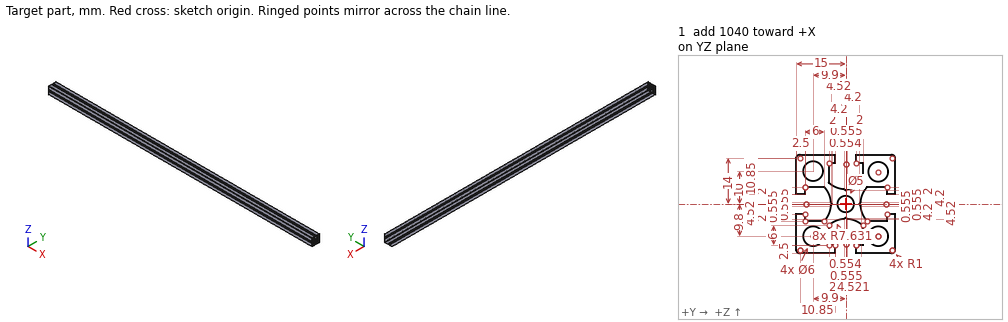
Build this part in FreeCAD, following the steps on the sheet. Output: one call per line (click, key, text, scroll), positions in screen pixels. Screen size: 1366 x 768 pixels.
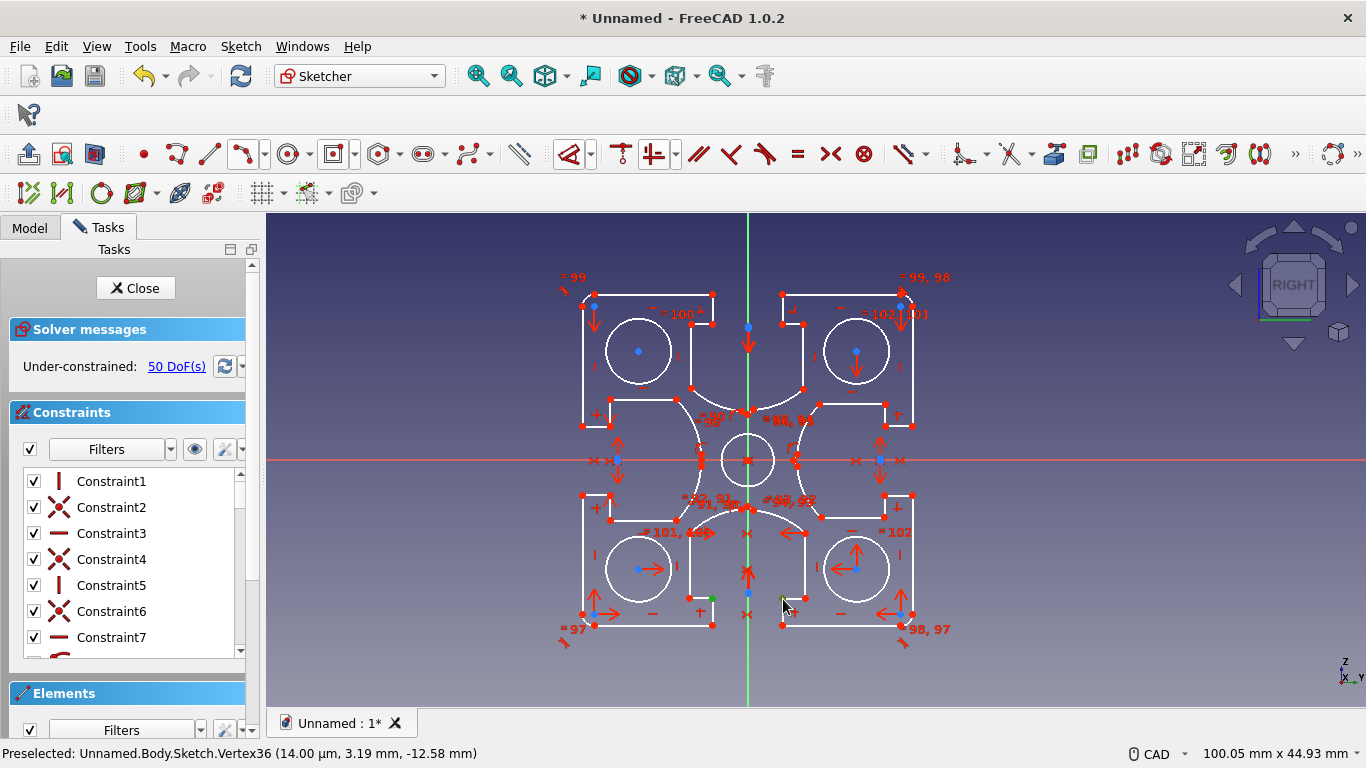
click(748, 648)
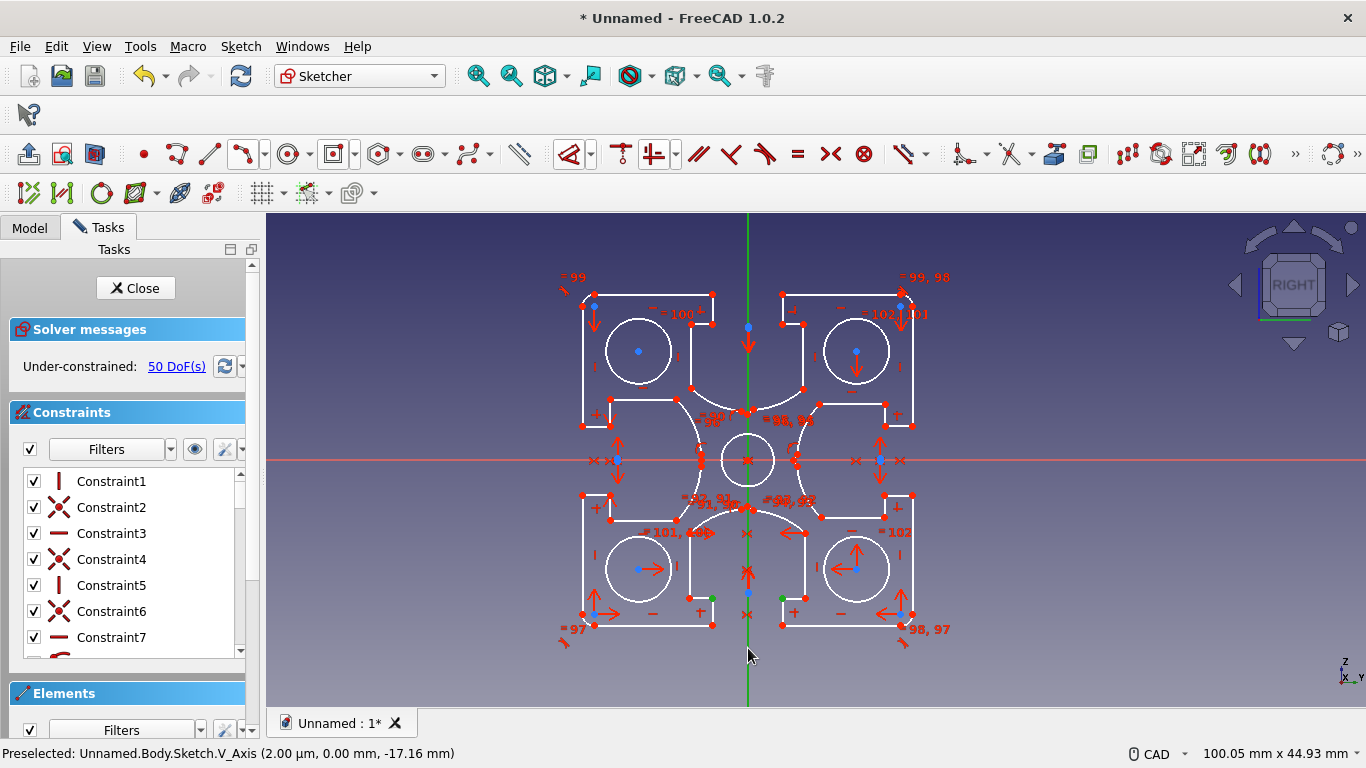
key(s)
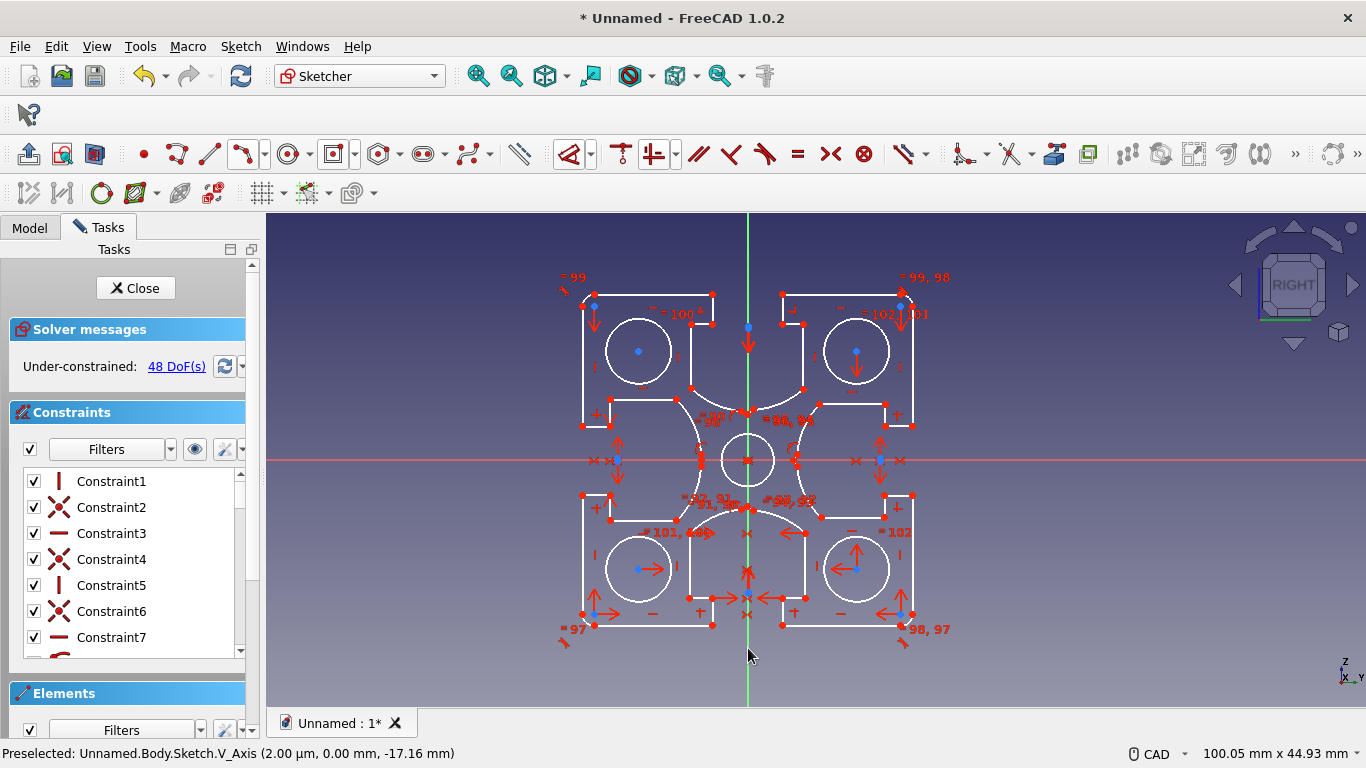
click(610, 495)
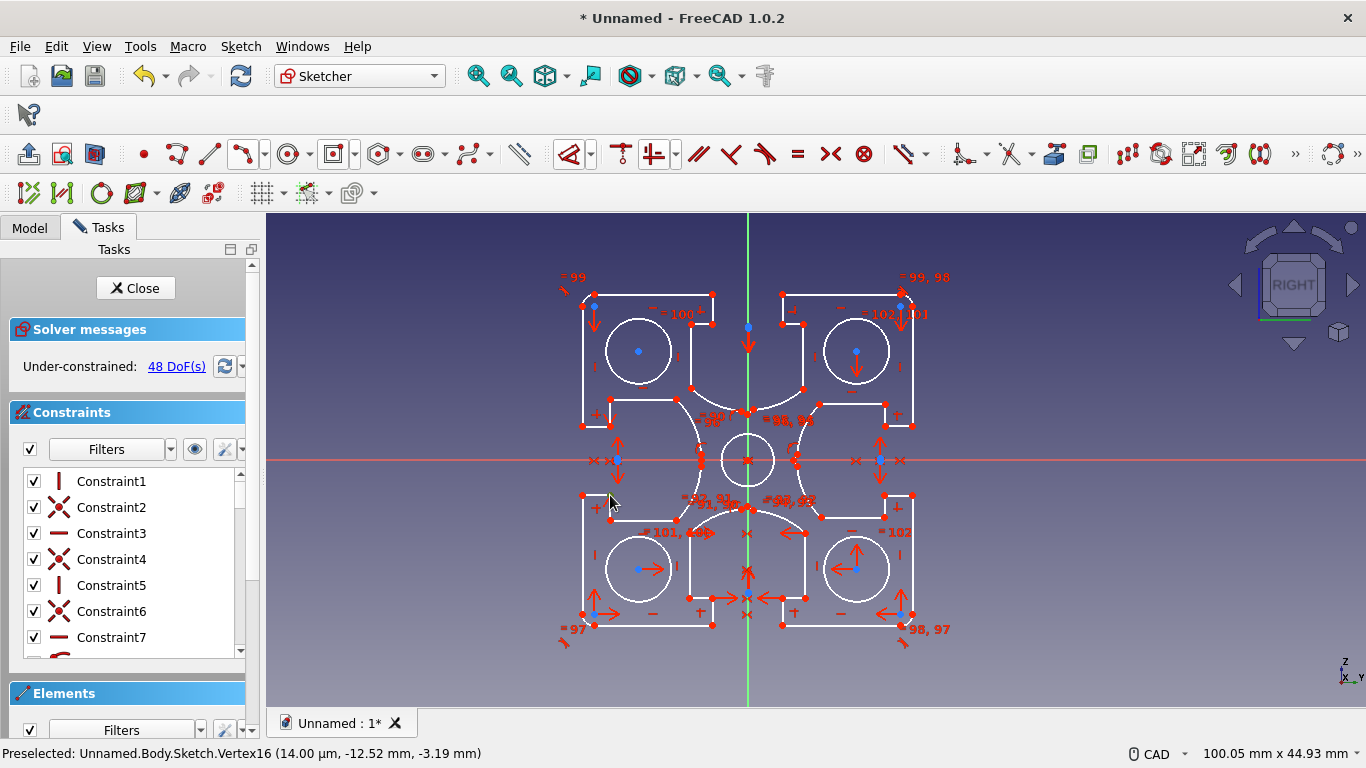
click(885, 496)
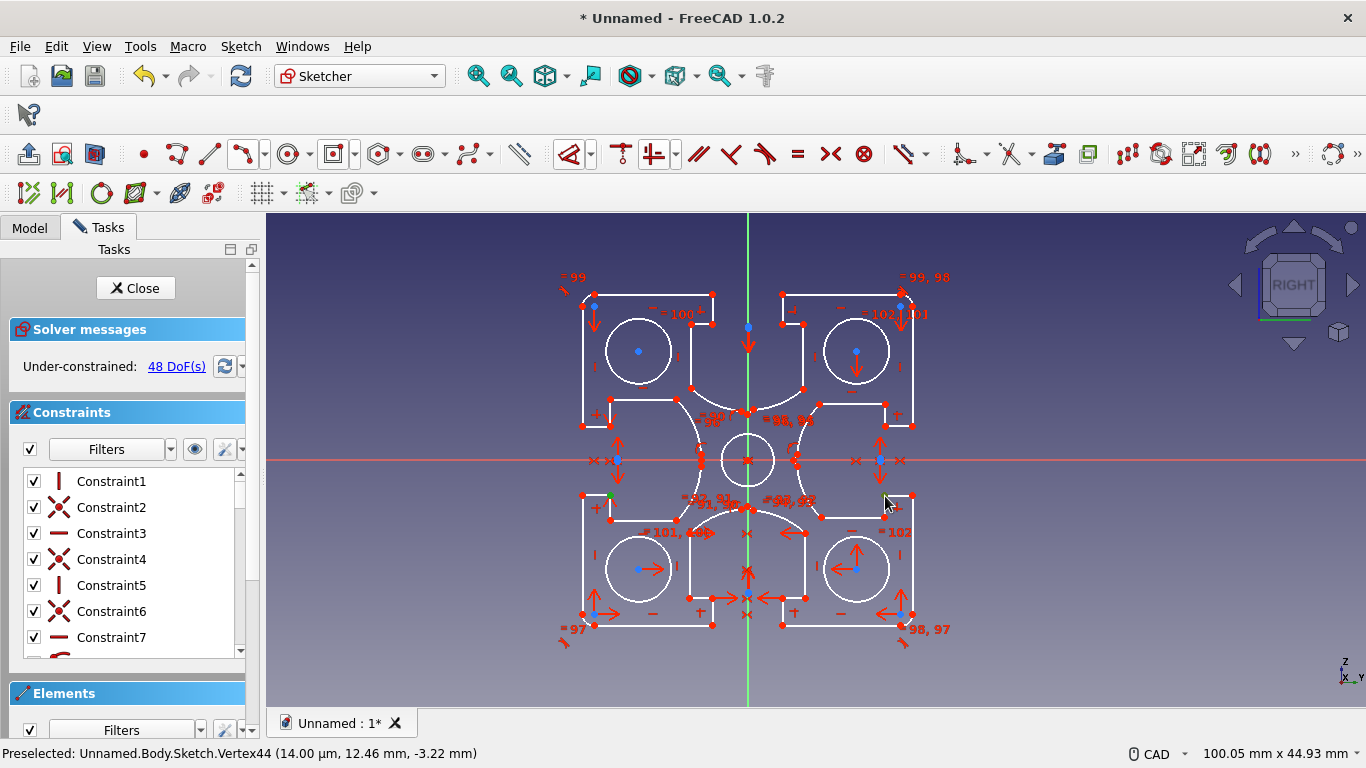
click(748, 648)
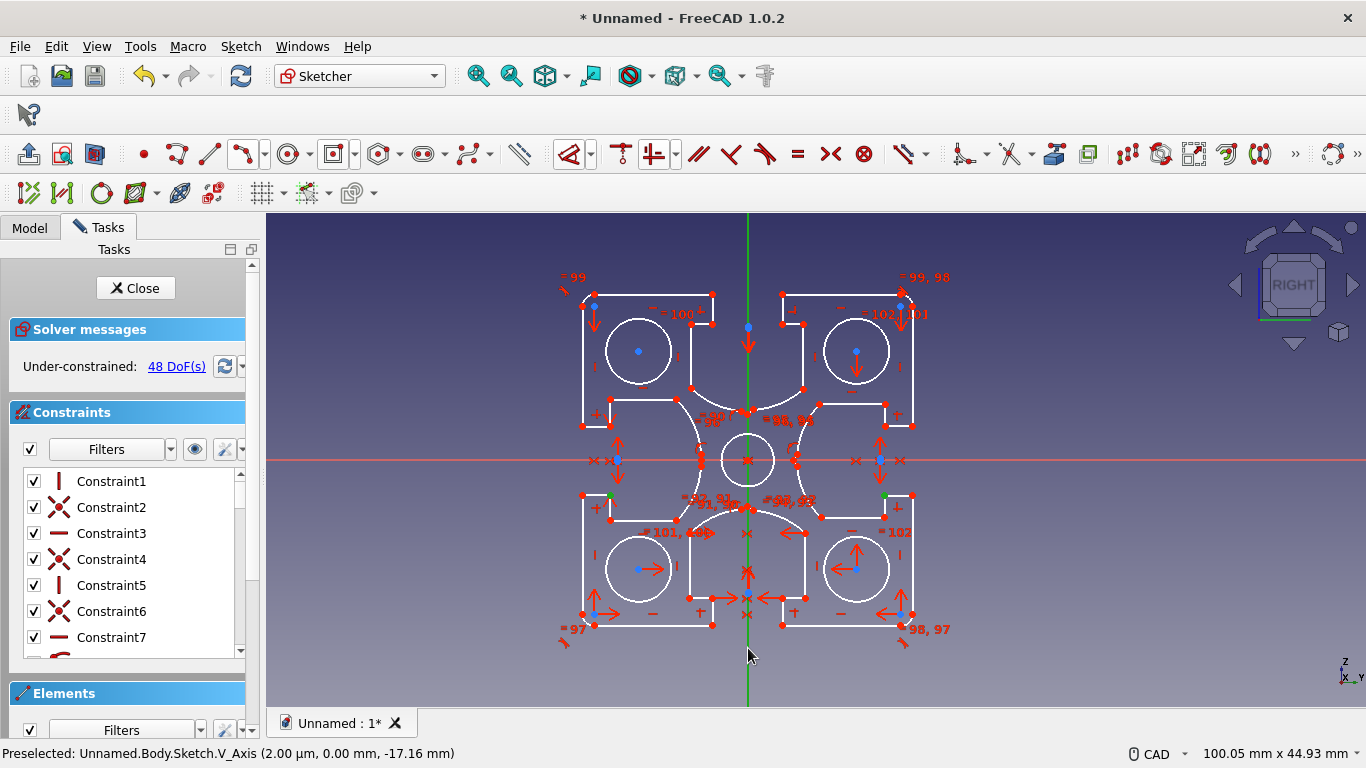
click(831, 154)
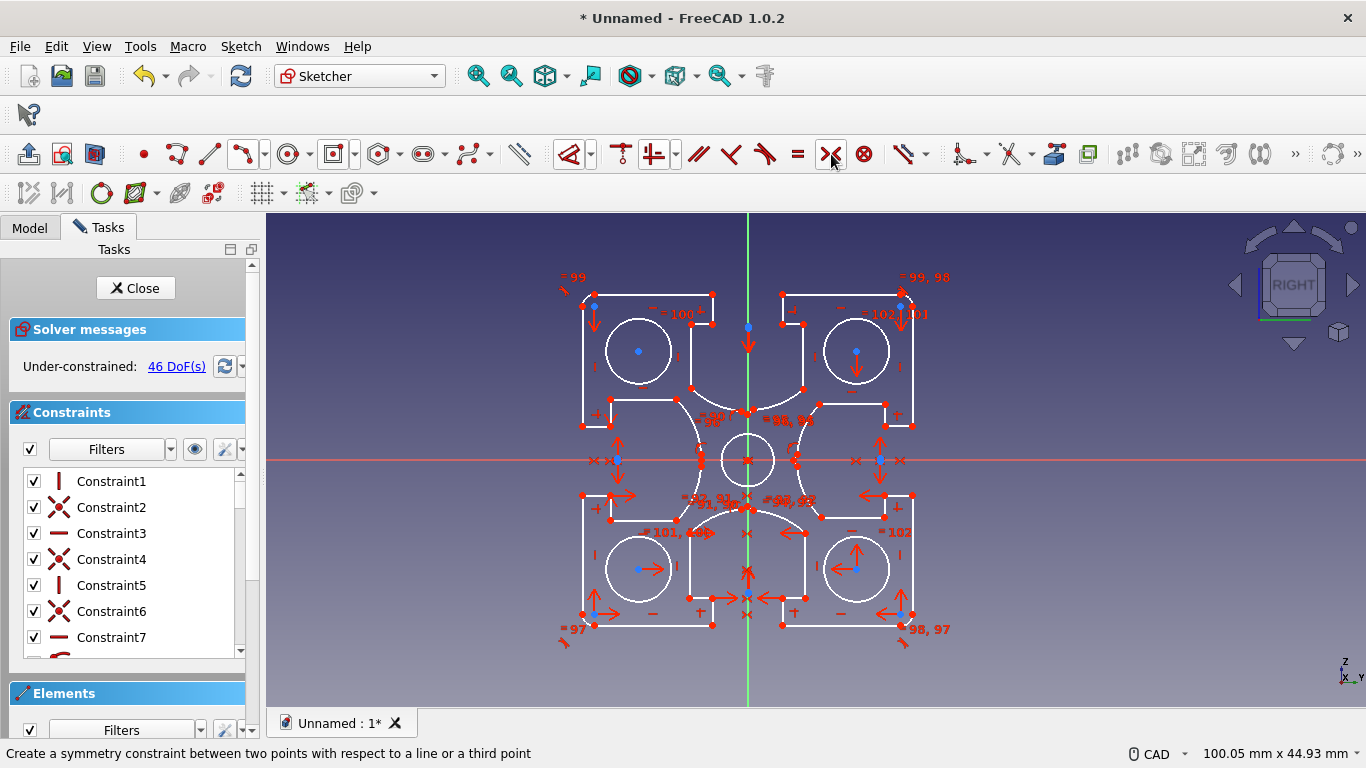
click(677, 521)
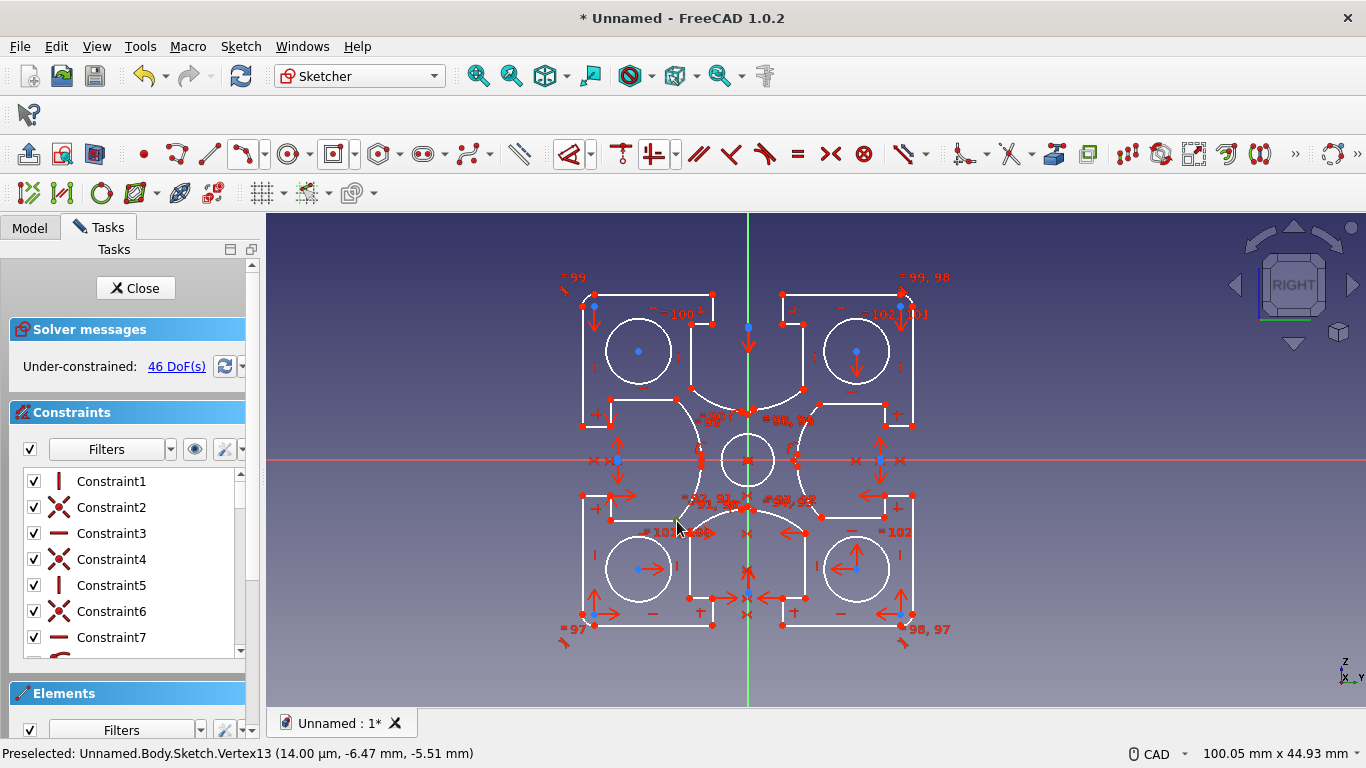
click(821, 518)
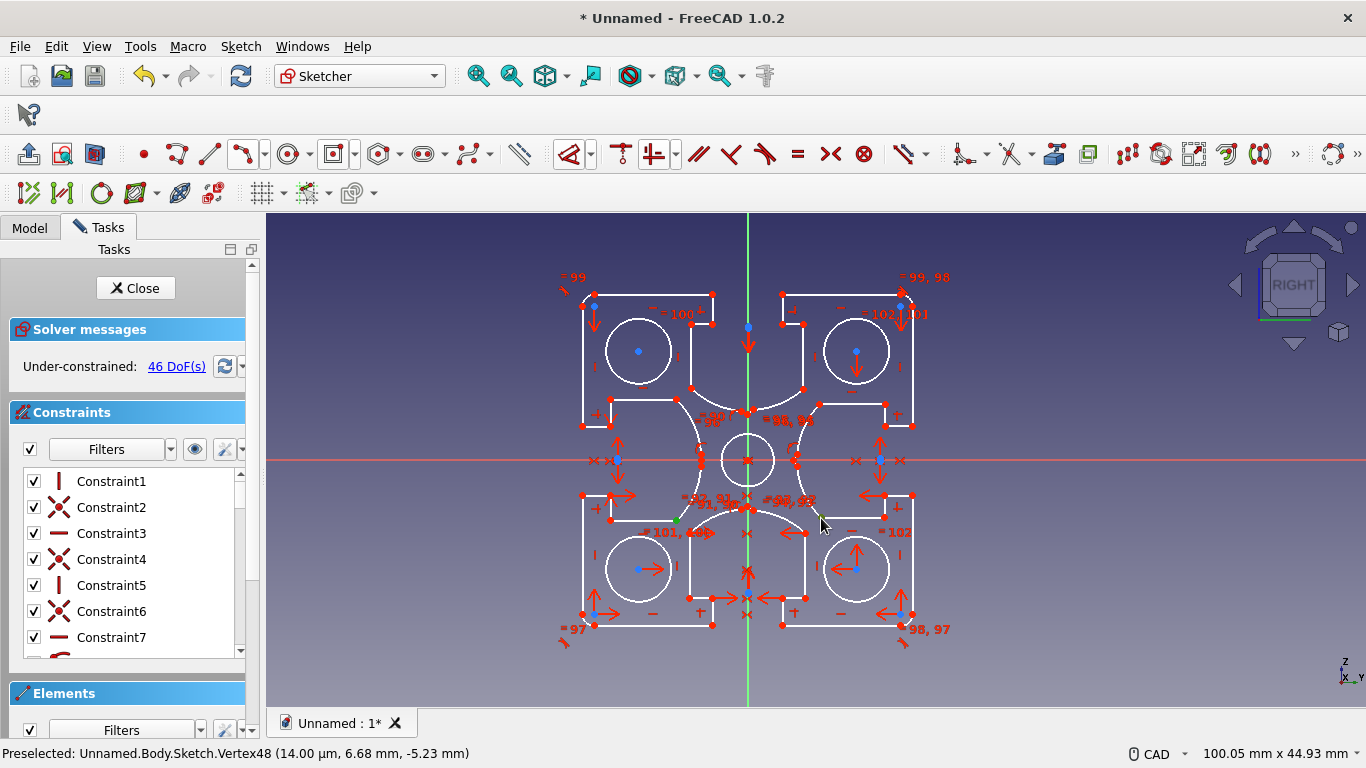
click(748, 648)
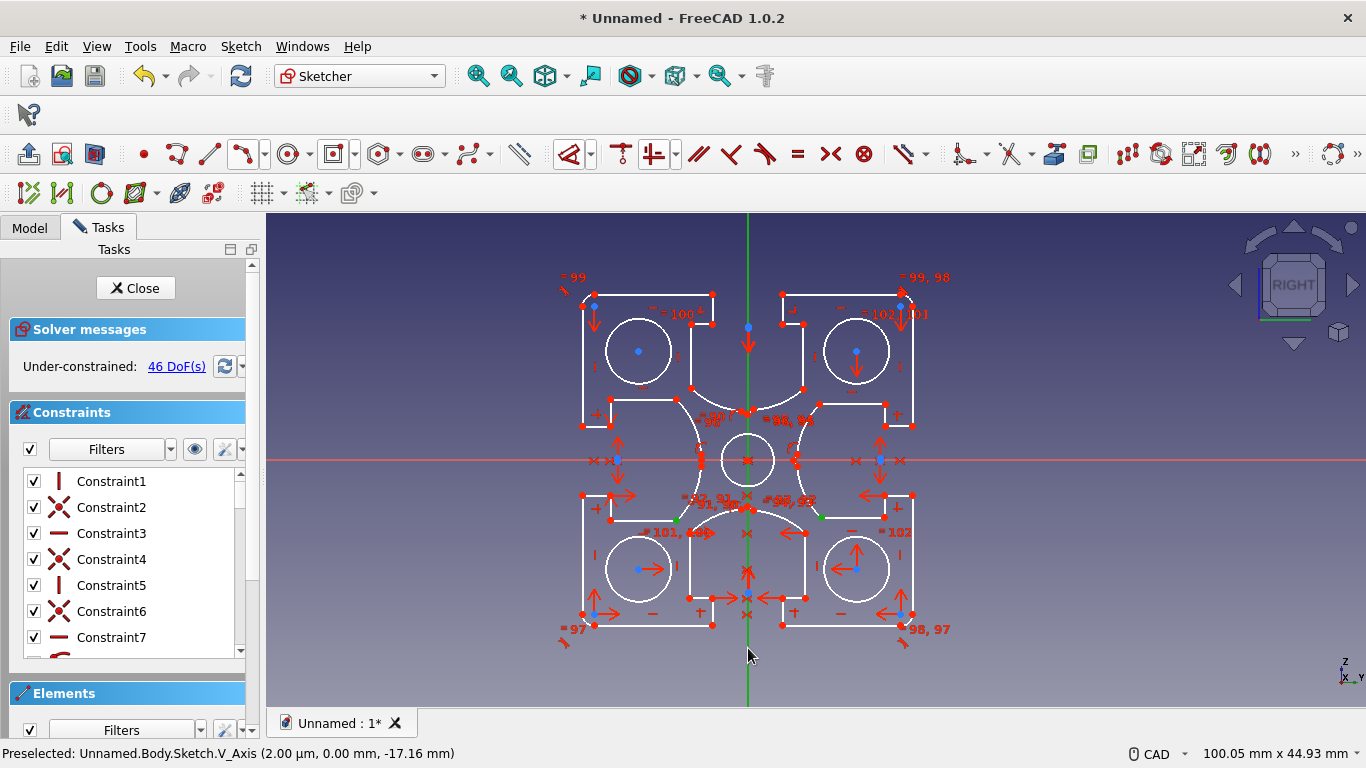
key(s)